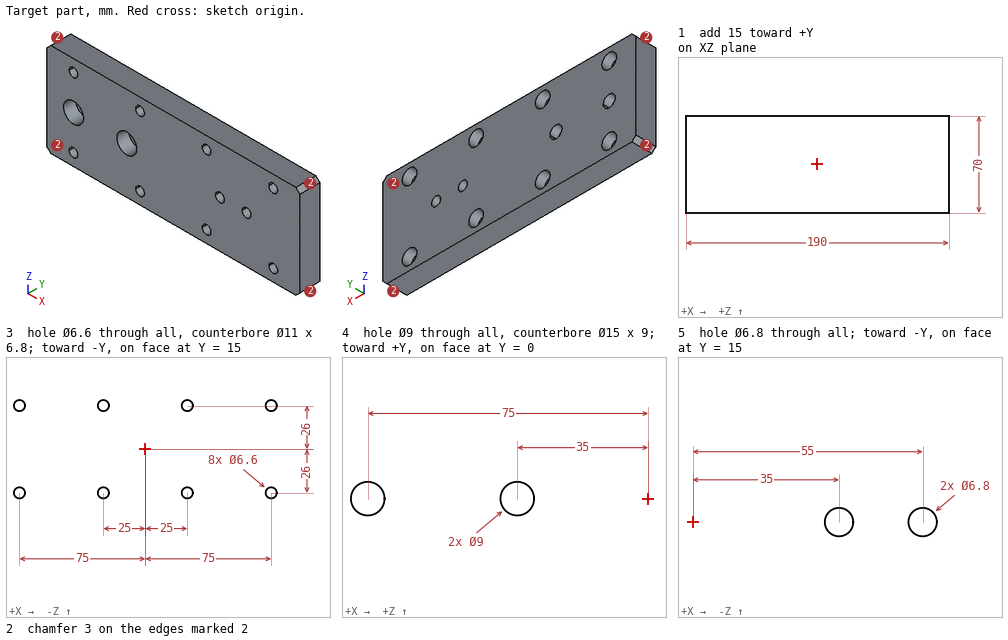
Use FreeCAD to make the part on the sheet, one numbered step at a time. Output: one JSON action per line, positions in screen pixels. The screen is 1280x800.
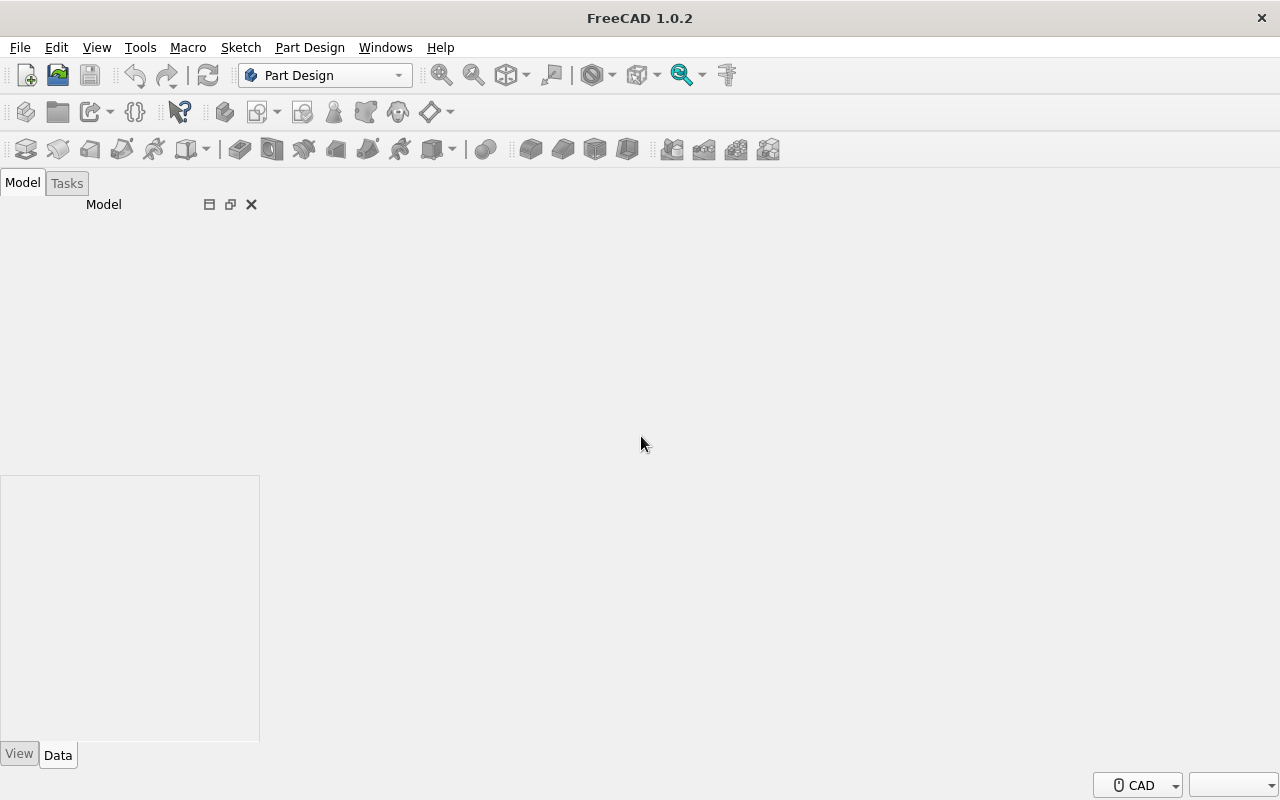
{"action": "key", "text": "ctrl+n"}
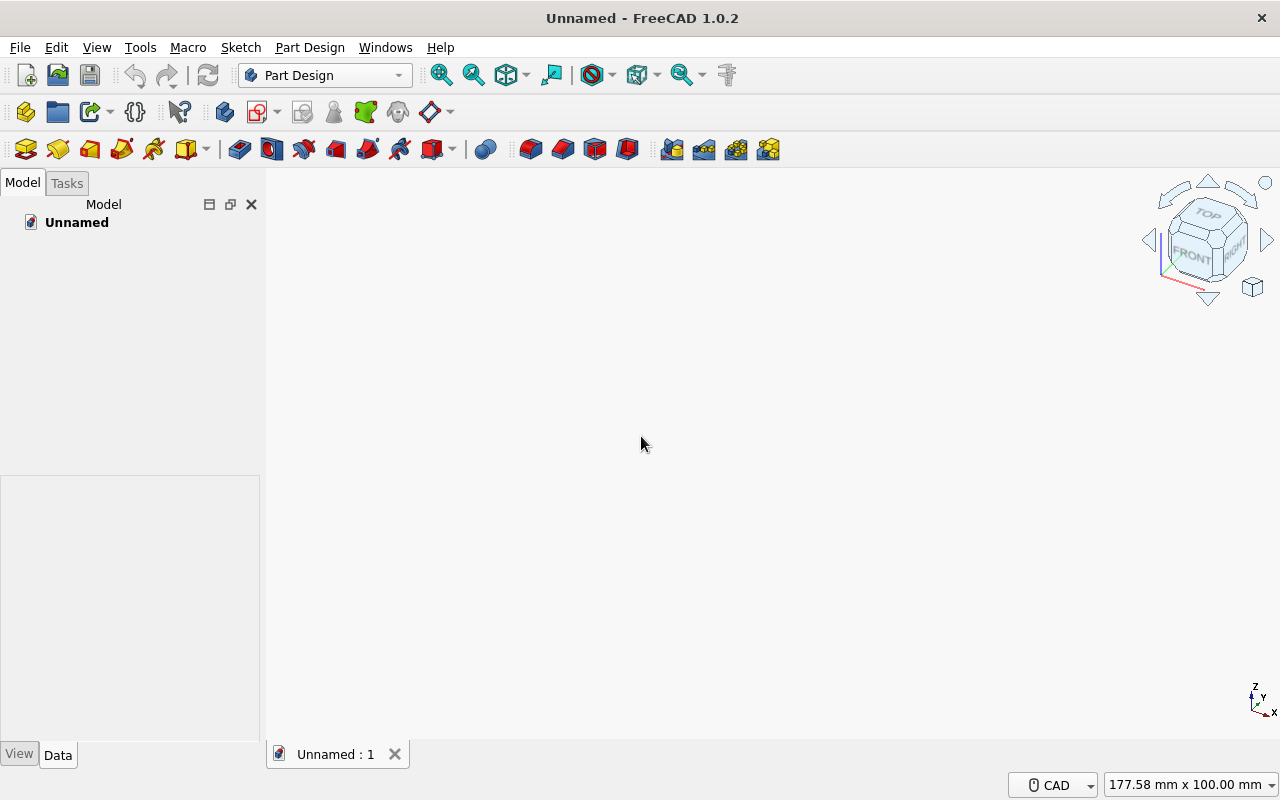
{"action": "left_click", "coordinate": [258, 112]}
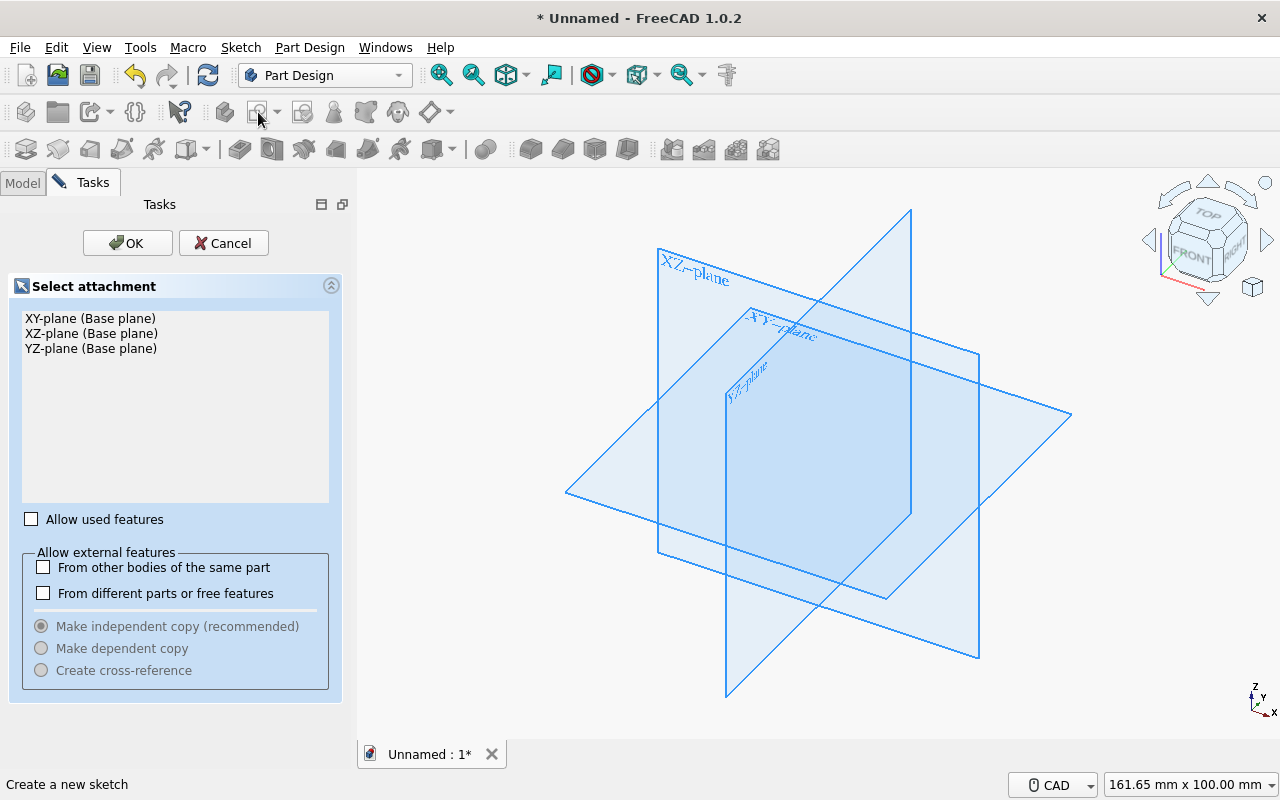
{"action": "left_click", "coordinate": [82, 334]}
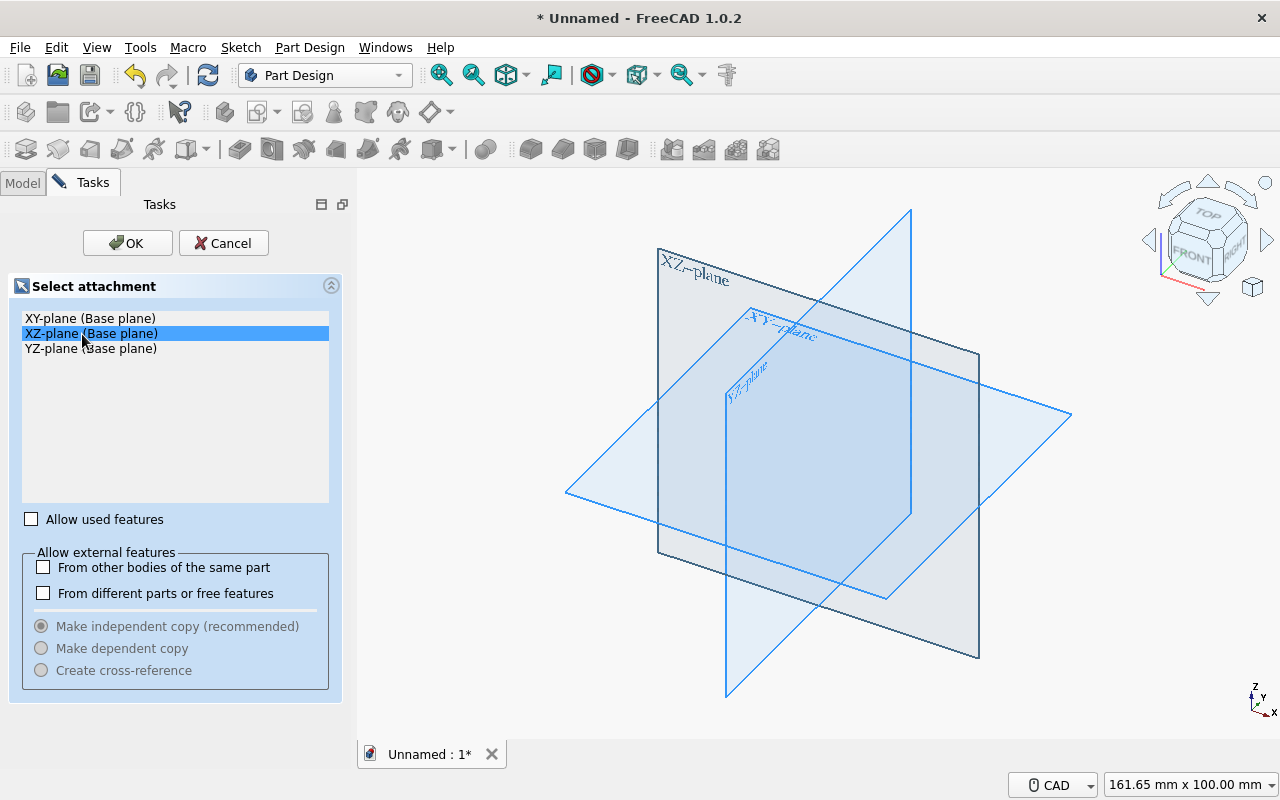
{"action": "left_click", "coordinate": [128, 243]}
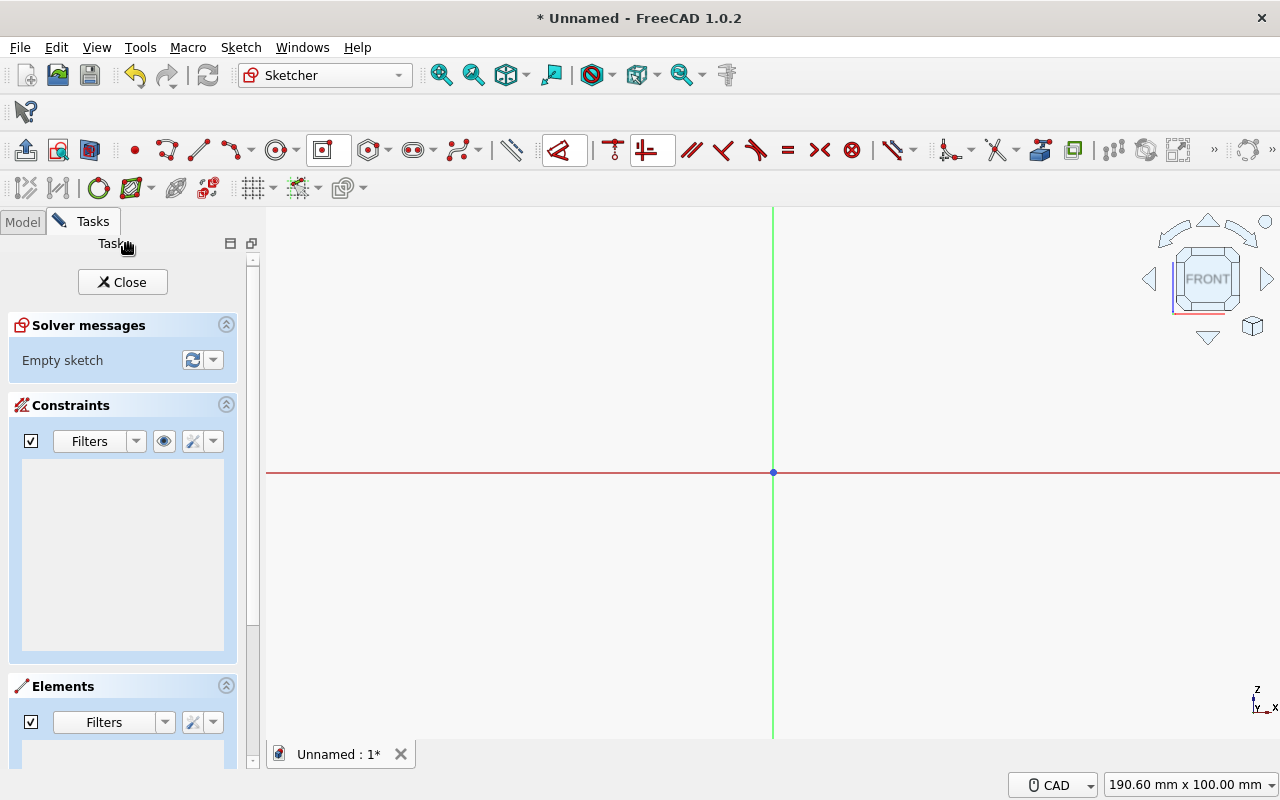
{"action": "scroll", "coordinate": [621, 473], "scroll_direction": "down", "scroll_amount": 3}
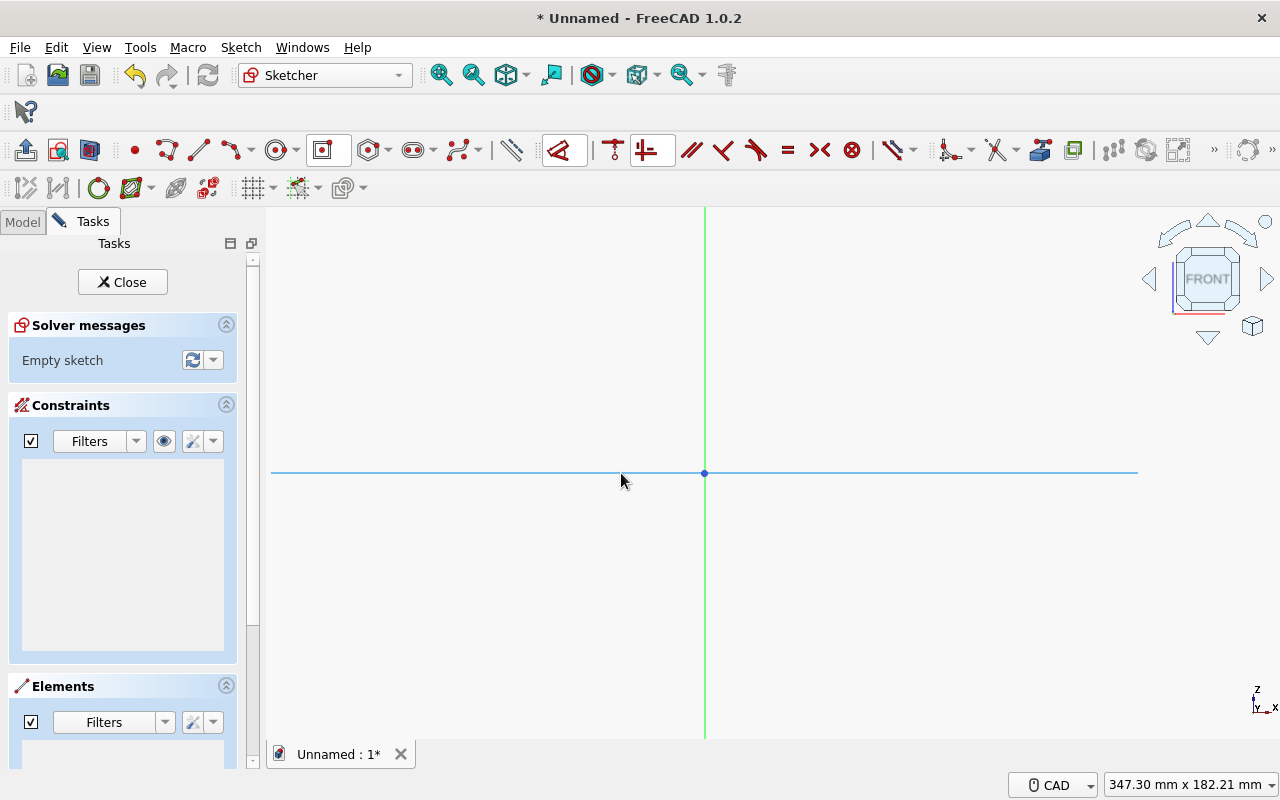
{"action": "key", "text": "g v"}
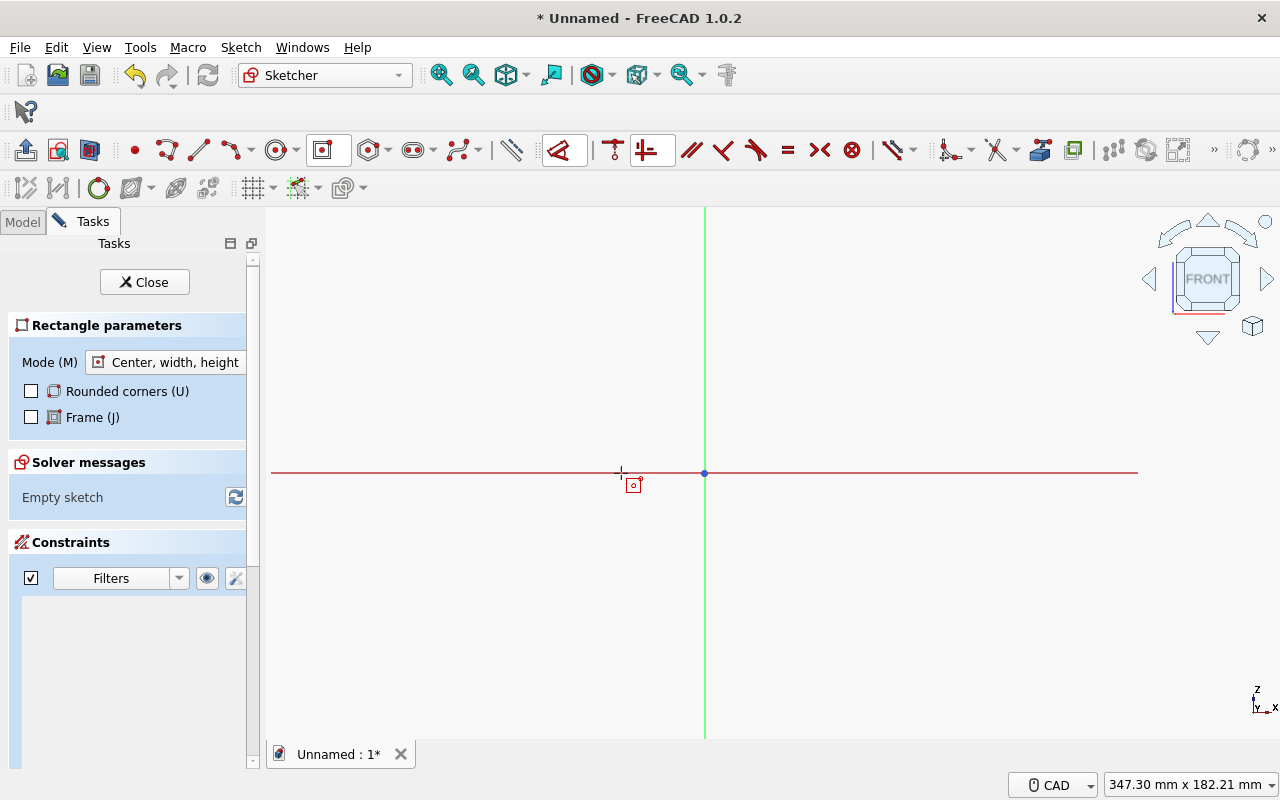
{"action": "left_click", "coordinate": [705, 473]}
{"action": "mouse_move", "coordinate": [982, 371]}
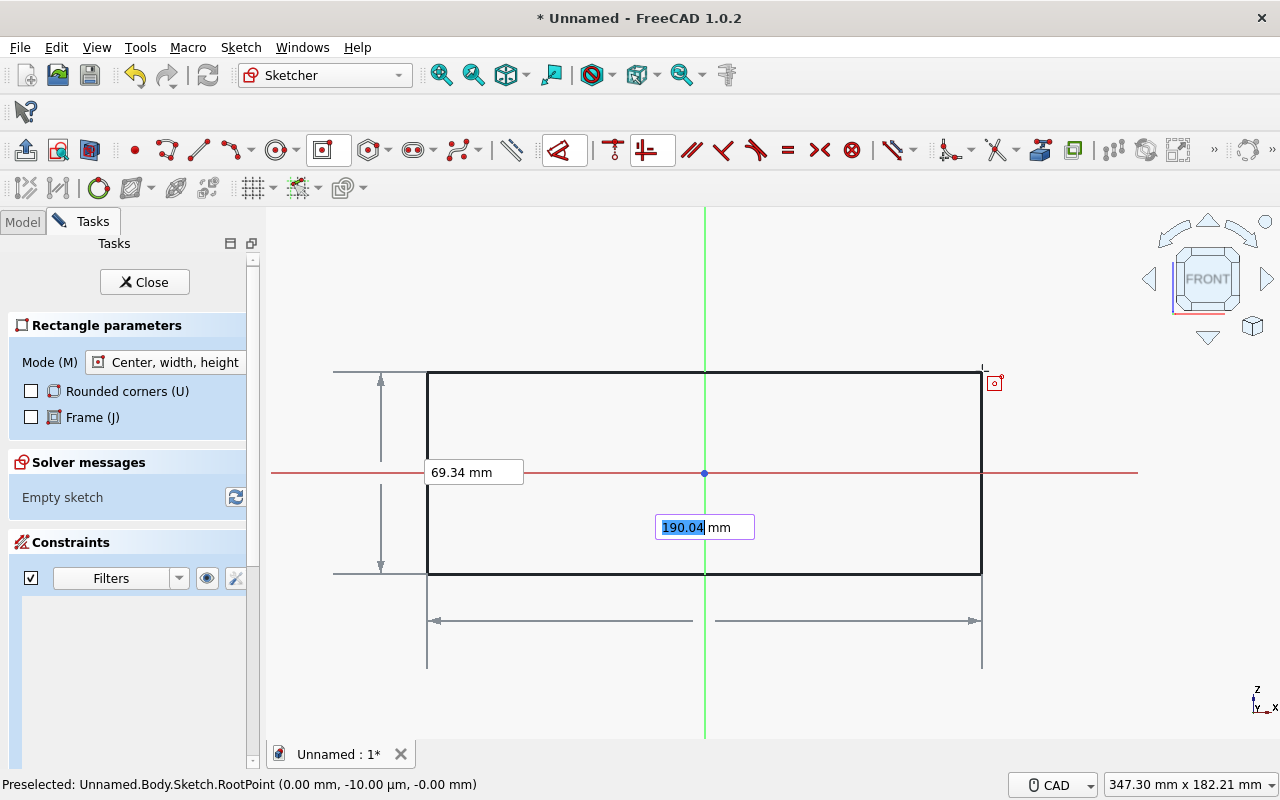
{"action": "type", "text": "190"}
{"action": "key", "text": "Tab"}
{"action": "type", "text": "70"}
{"action": "key", "text": "Return"}
{"action": "key", "text": "Escape"}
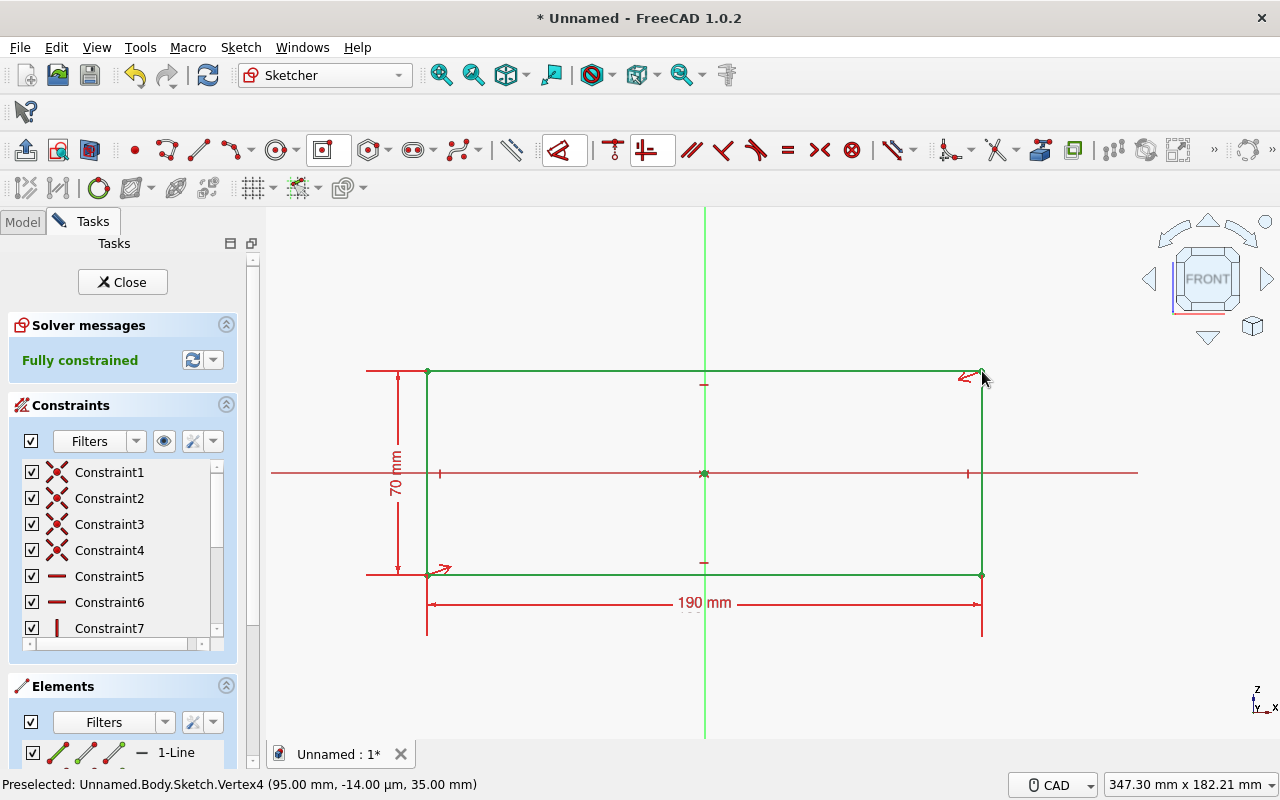
{"action": "left_click", "coordinate": [123, 282]}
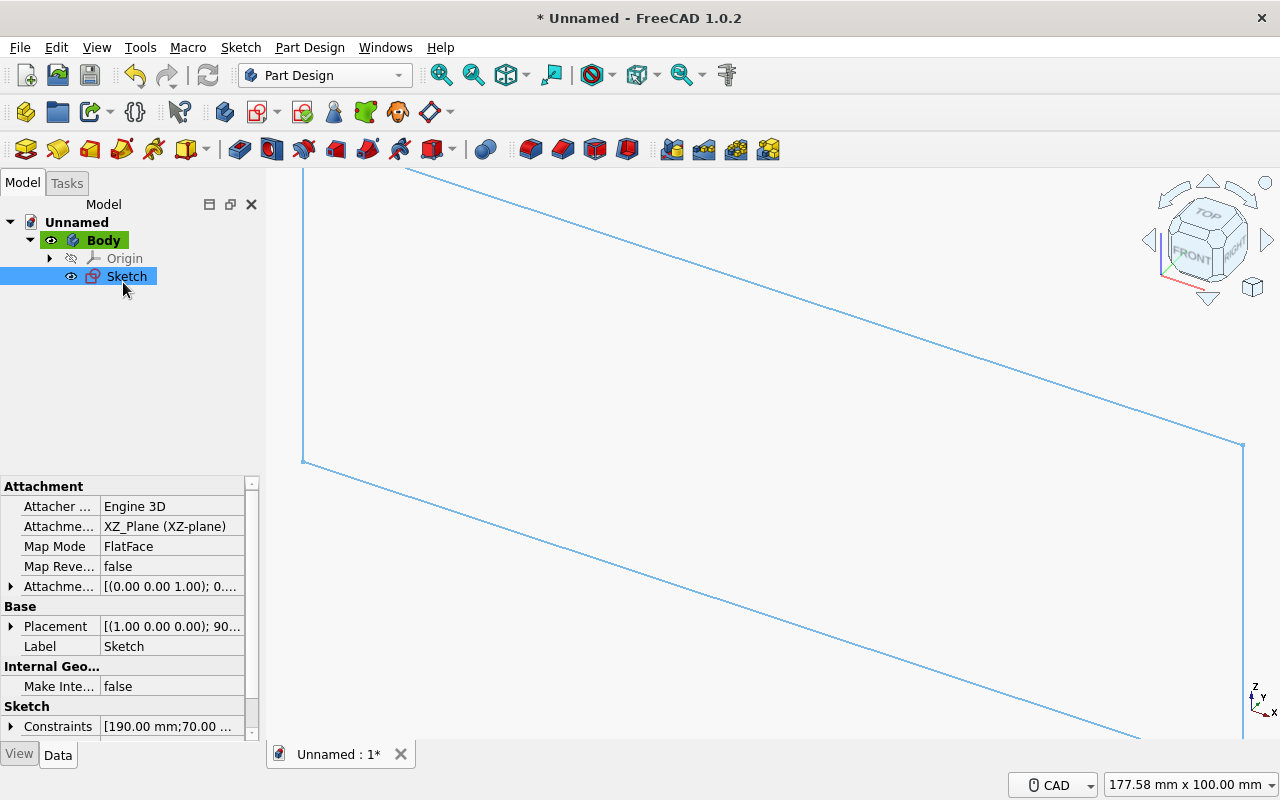
{"action": "left_click", "coordinate": [26, 150]}